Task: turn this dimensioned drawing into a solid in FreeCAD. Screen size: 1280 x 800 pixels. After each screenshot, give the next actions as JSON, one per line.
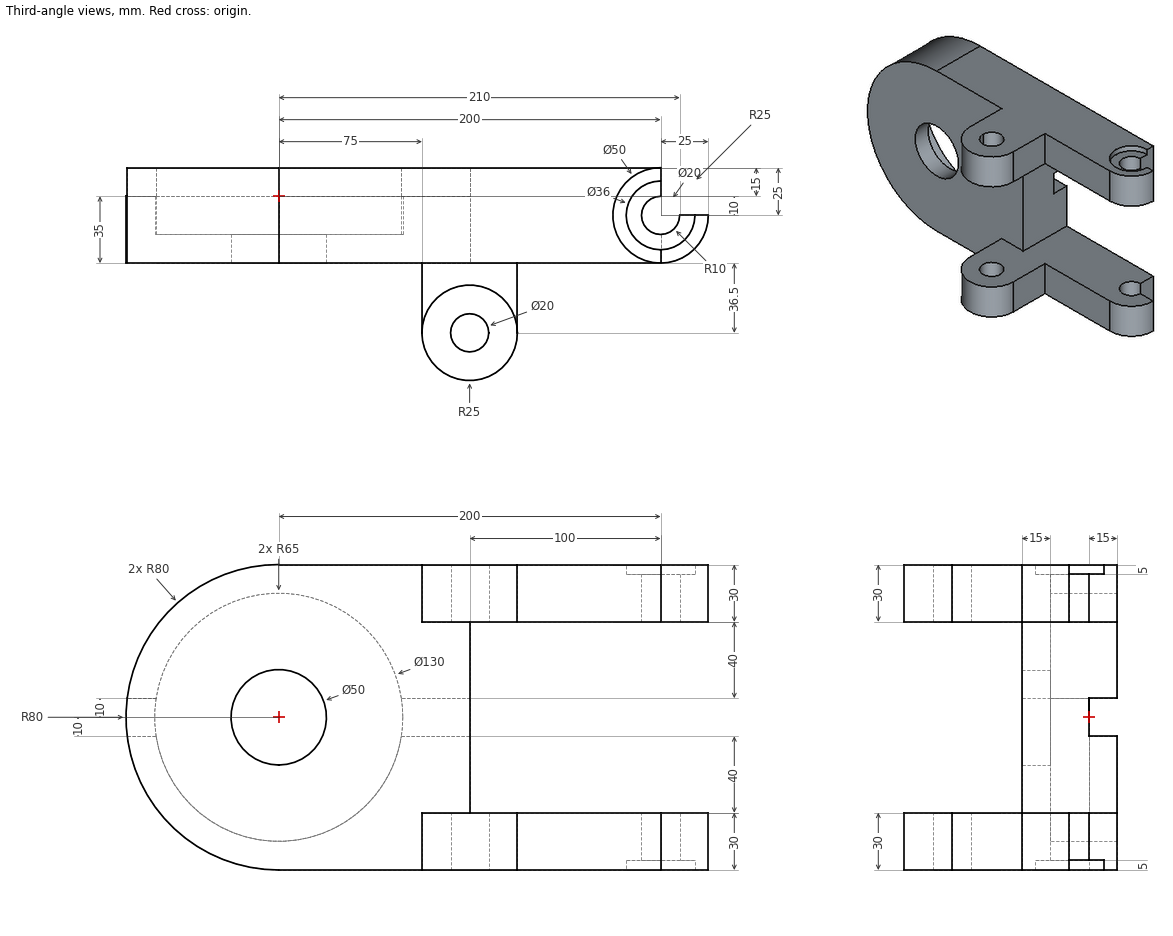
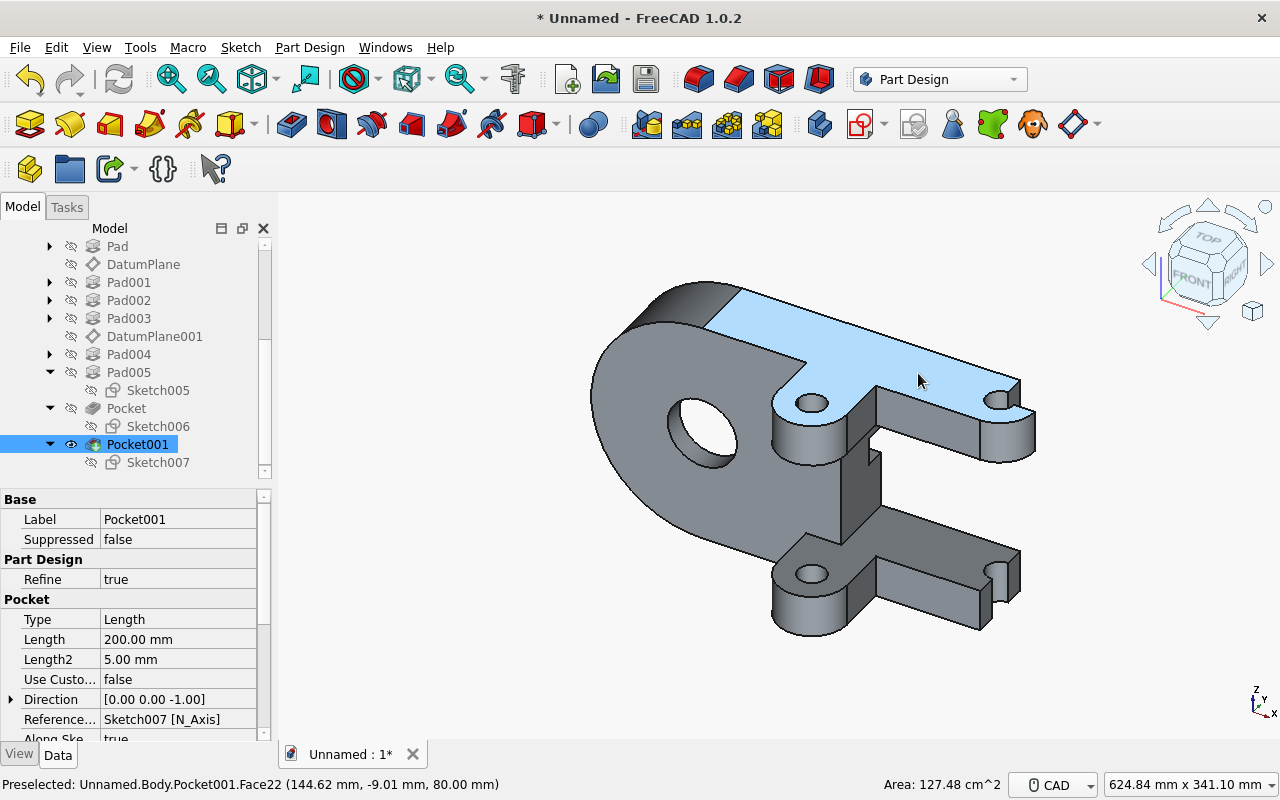
{"action": "left_click", "coordinate": [860, 124]}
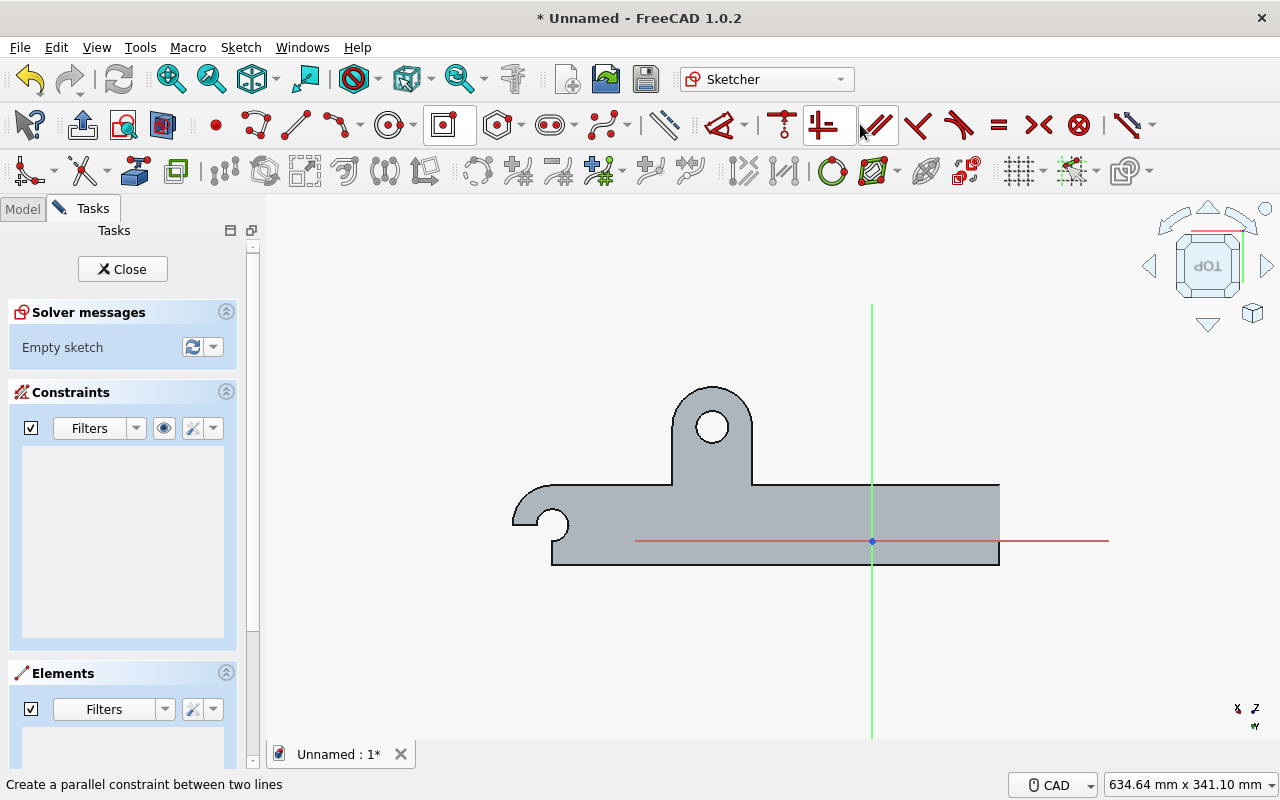
{"action": "scroll", "coordinate": [522, 537], "scroll_direction": "up", "scroll_amount": 9}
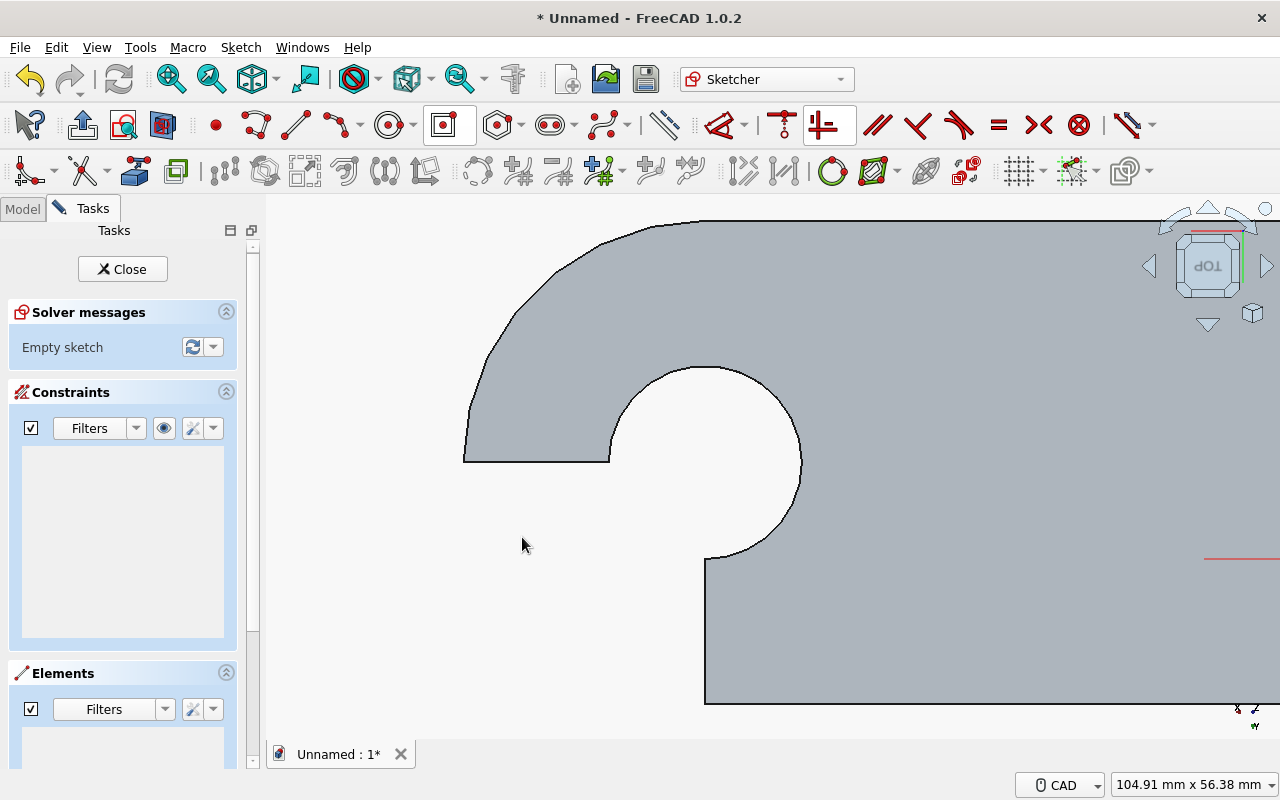
{"action": "left_click", "coordinate": [390, 126]}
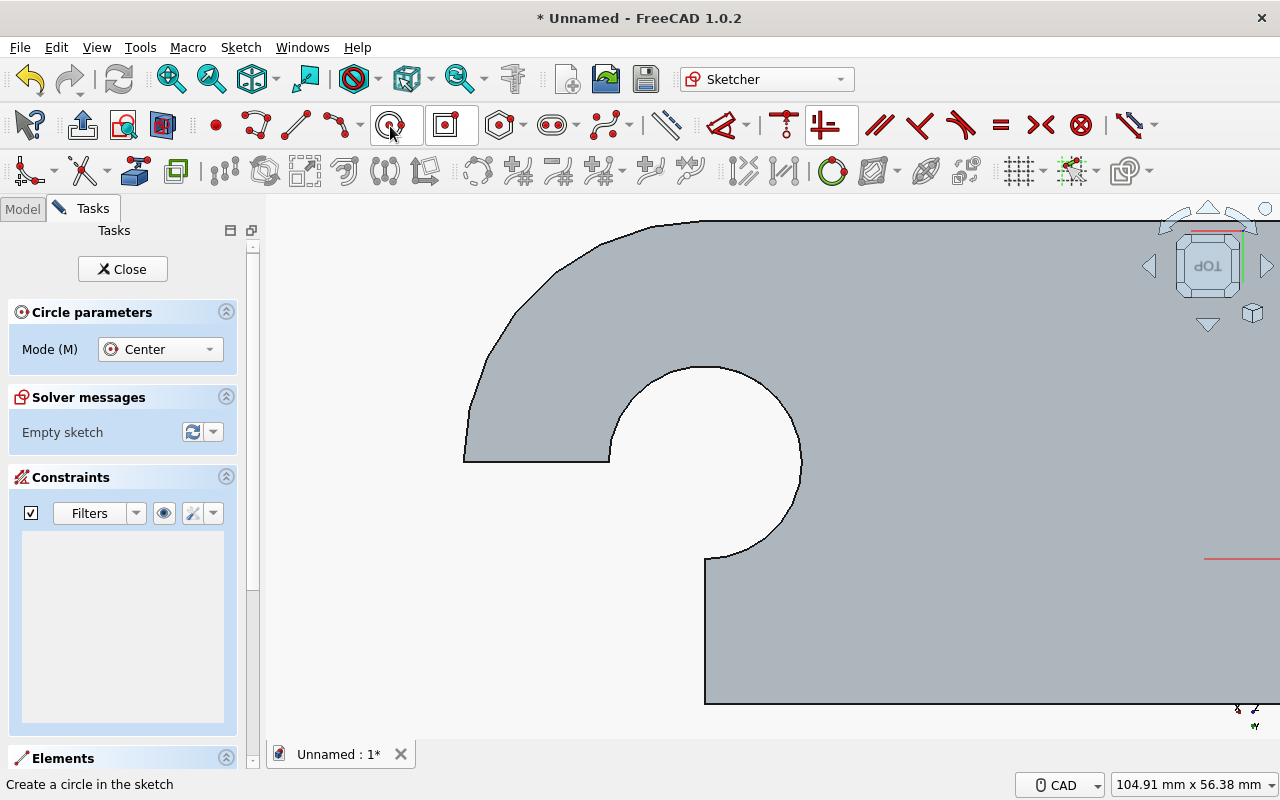
{"action": "left_click", "coordinate": [705, 462]}
{"action": "left_click", "coordinate": [828, 339]}
{"action": "key", "text": "Escape"}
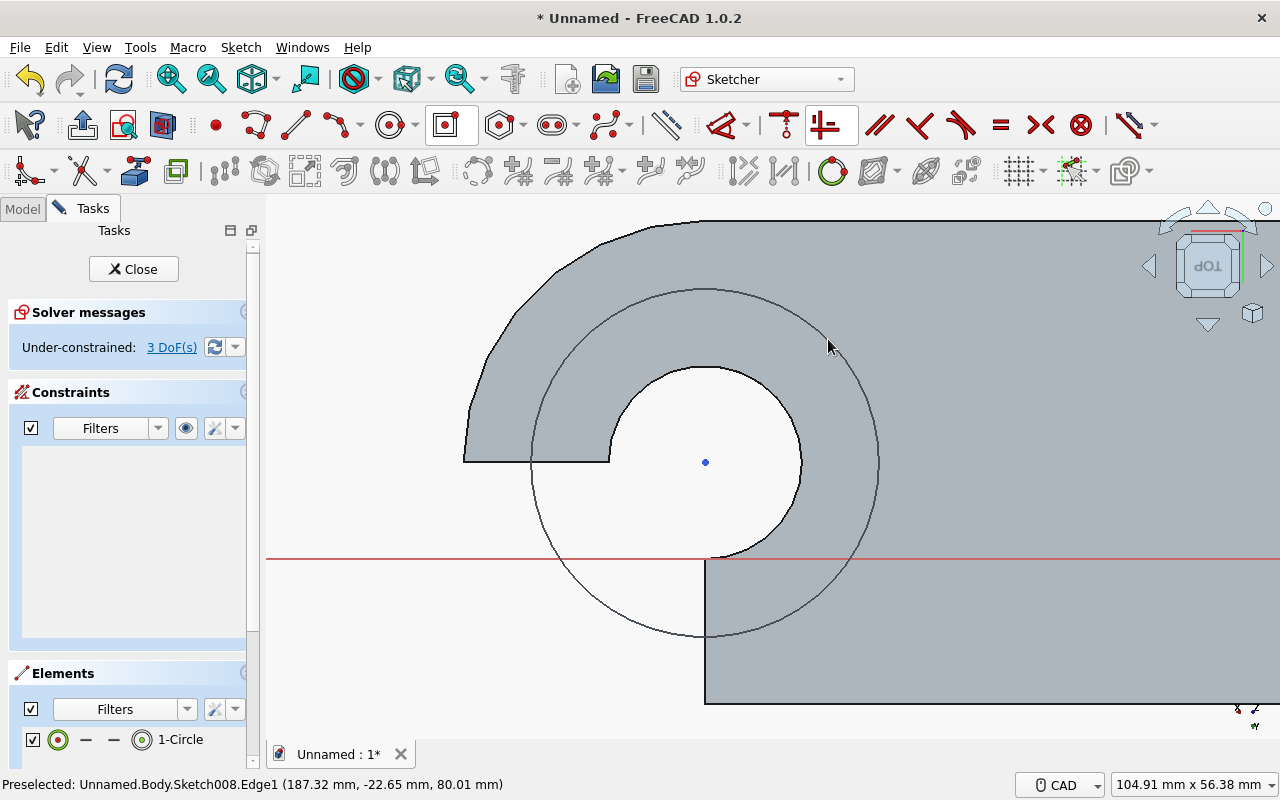
{"action": "left_click", "coordinate": [722, 126]}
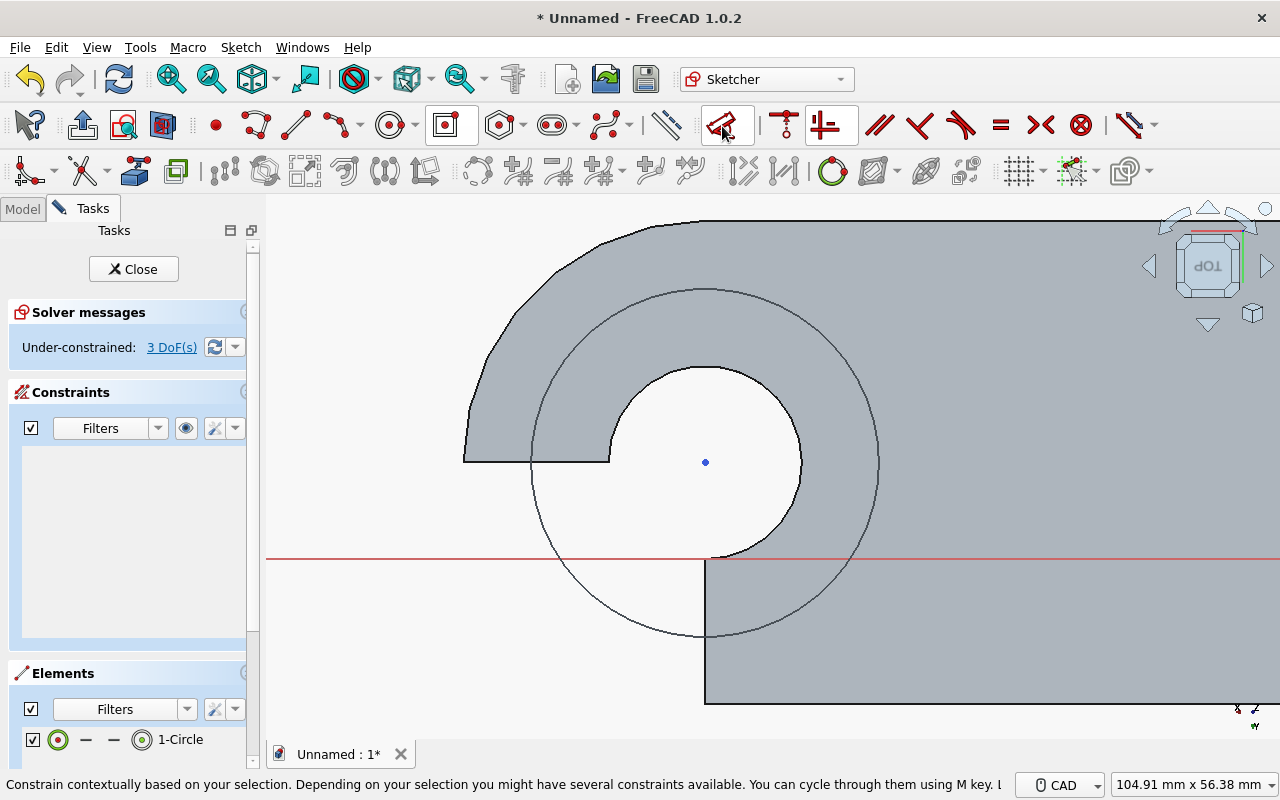
{"action": "left_click", "coordinate": [828, 340]}
{"action": "left_click", "coordinate": [851, 317]}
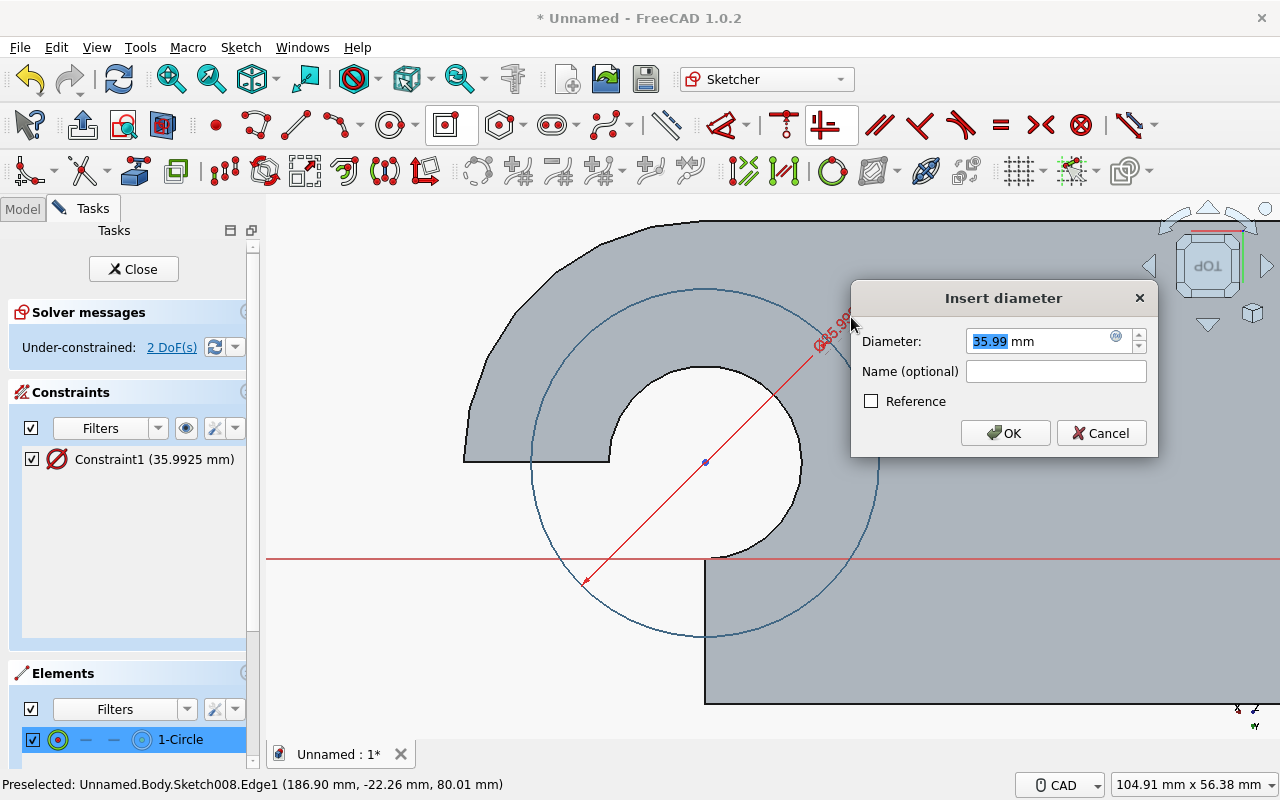
{"action": "type", "text": "36"}
{"action": "key", "text": "Return"}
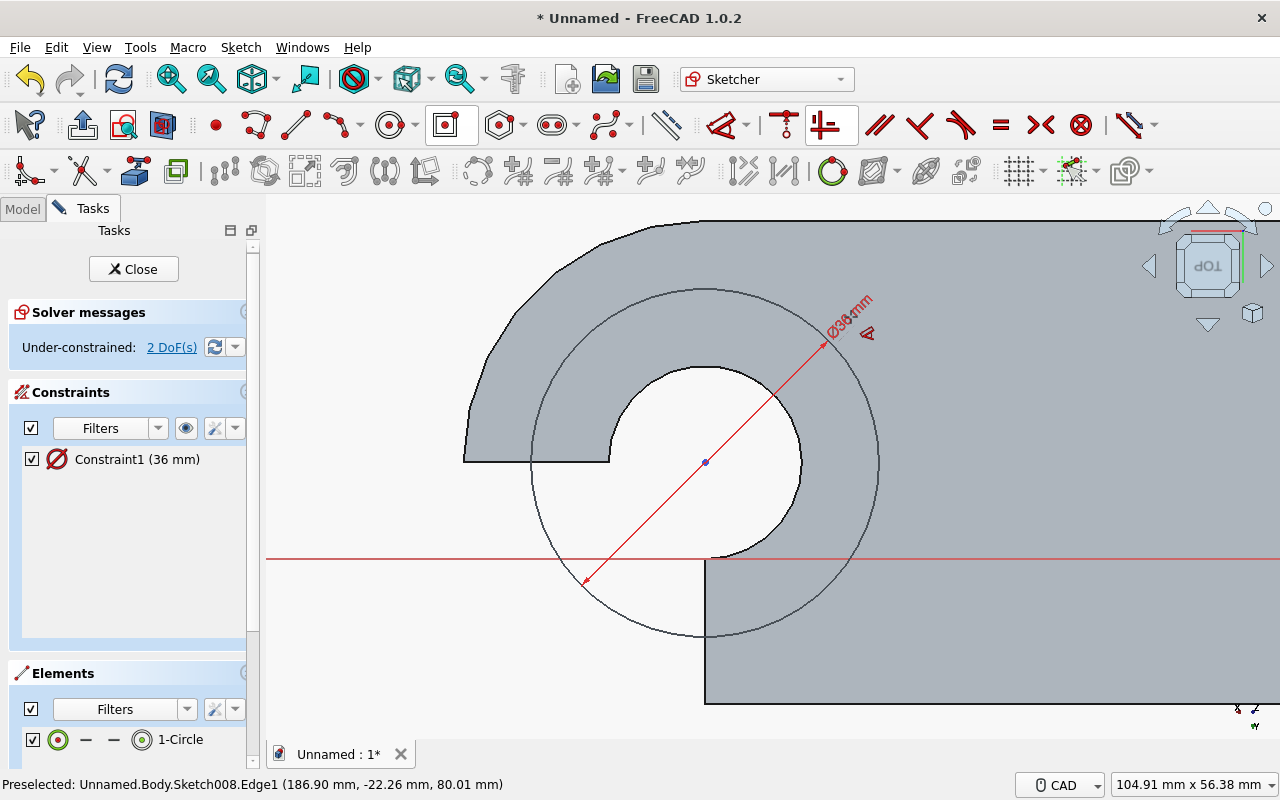
{"action": "left_click", "coordinate": [705, 463]}
{"action": "left_click", "coordinate": [671, 511]}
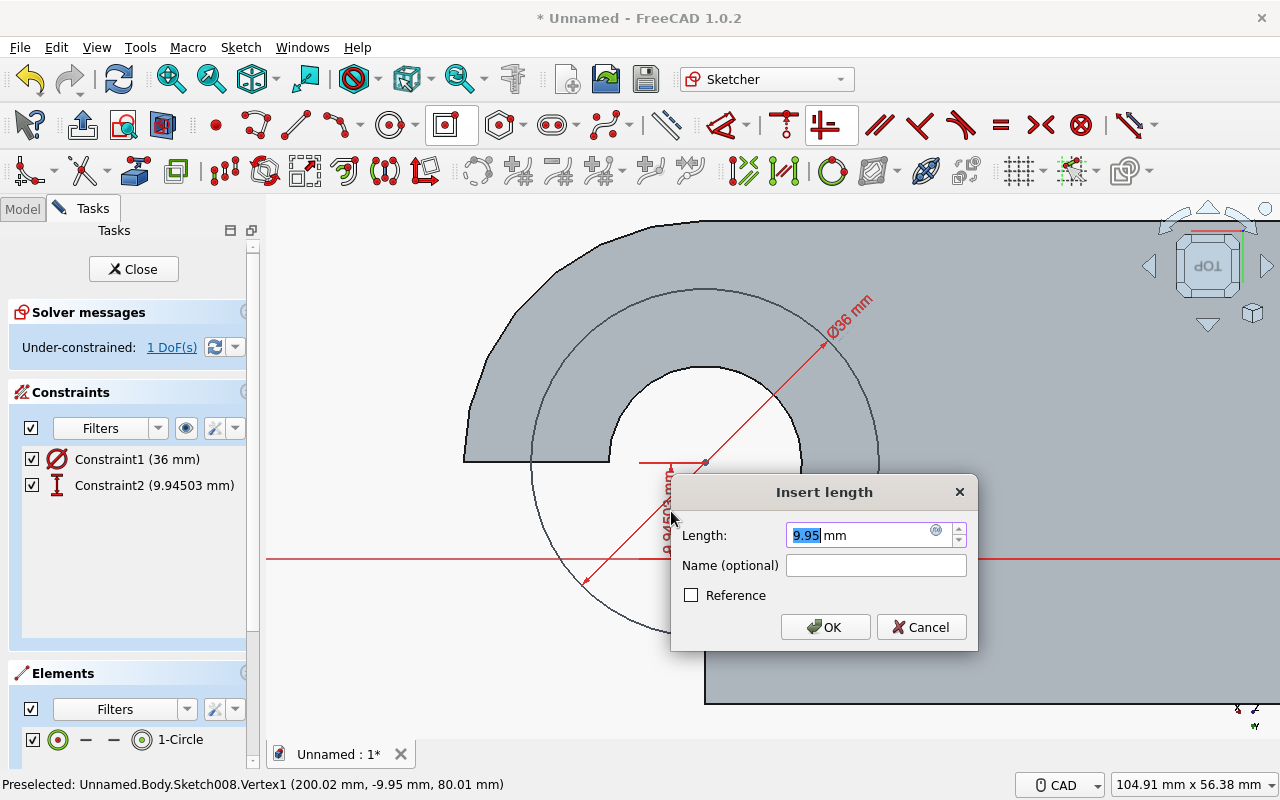
{"action": "type", "text": "10"}
{"action": "key", "text": "Return"}